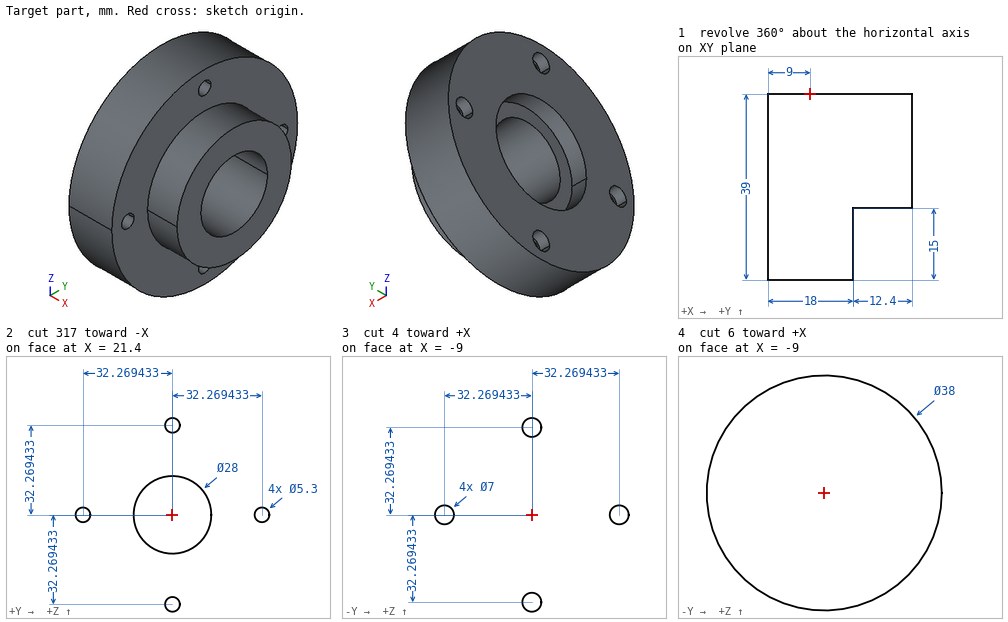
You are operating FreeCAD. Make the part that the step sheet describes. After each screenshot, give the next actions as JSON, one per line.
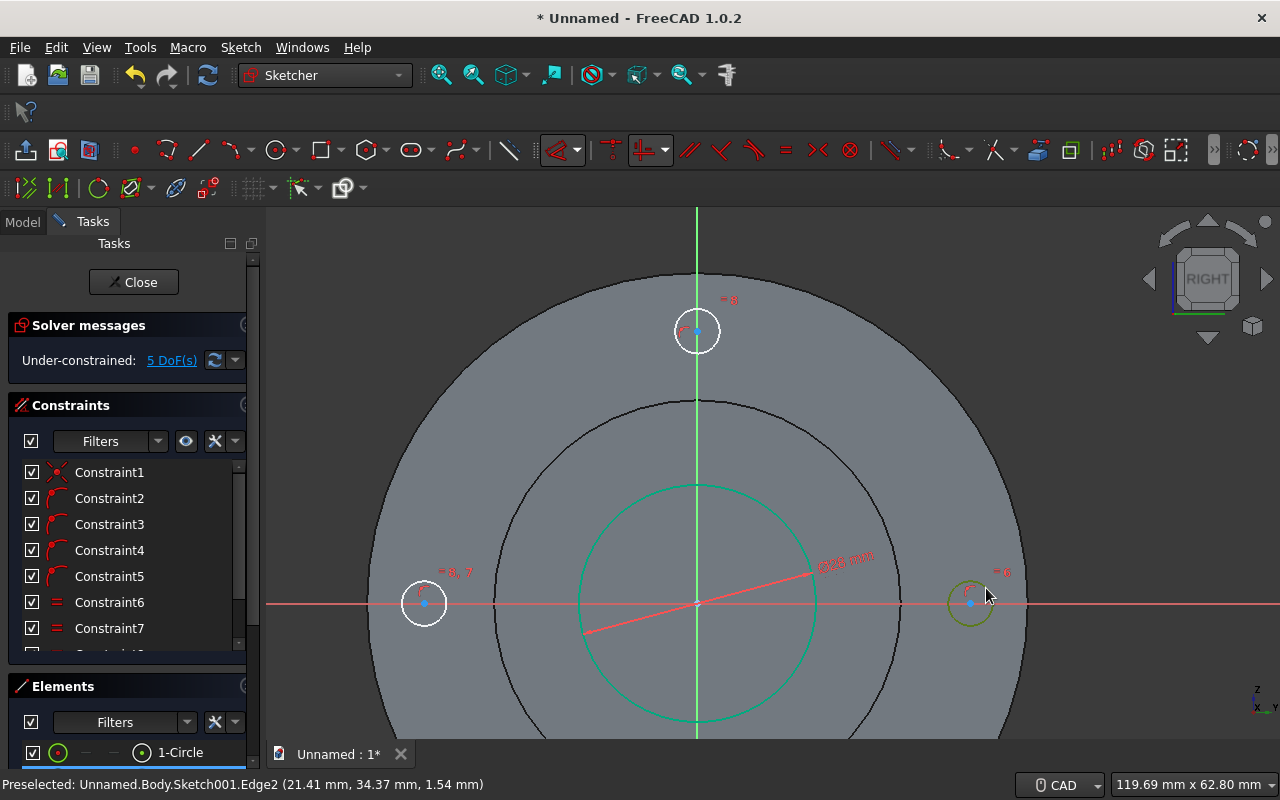
{"action": "key", "text": "k o"}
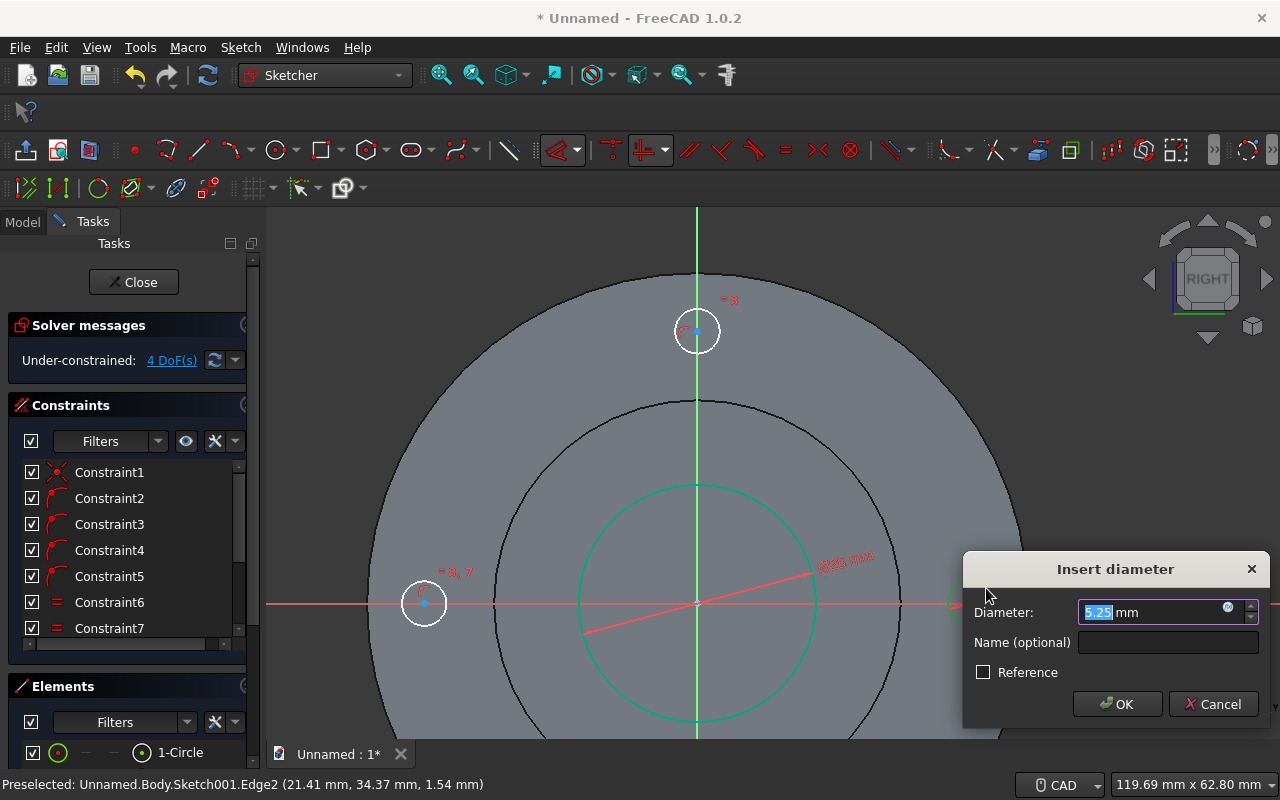
{"action": "type", "text": "5.3"}
{"action": "key", "text": "Return"}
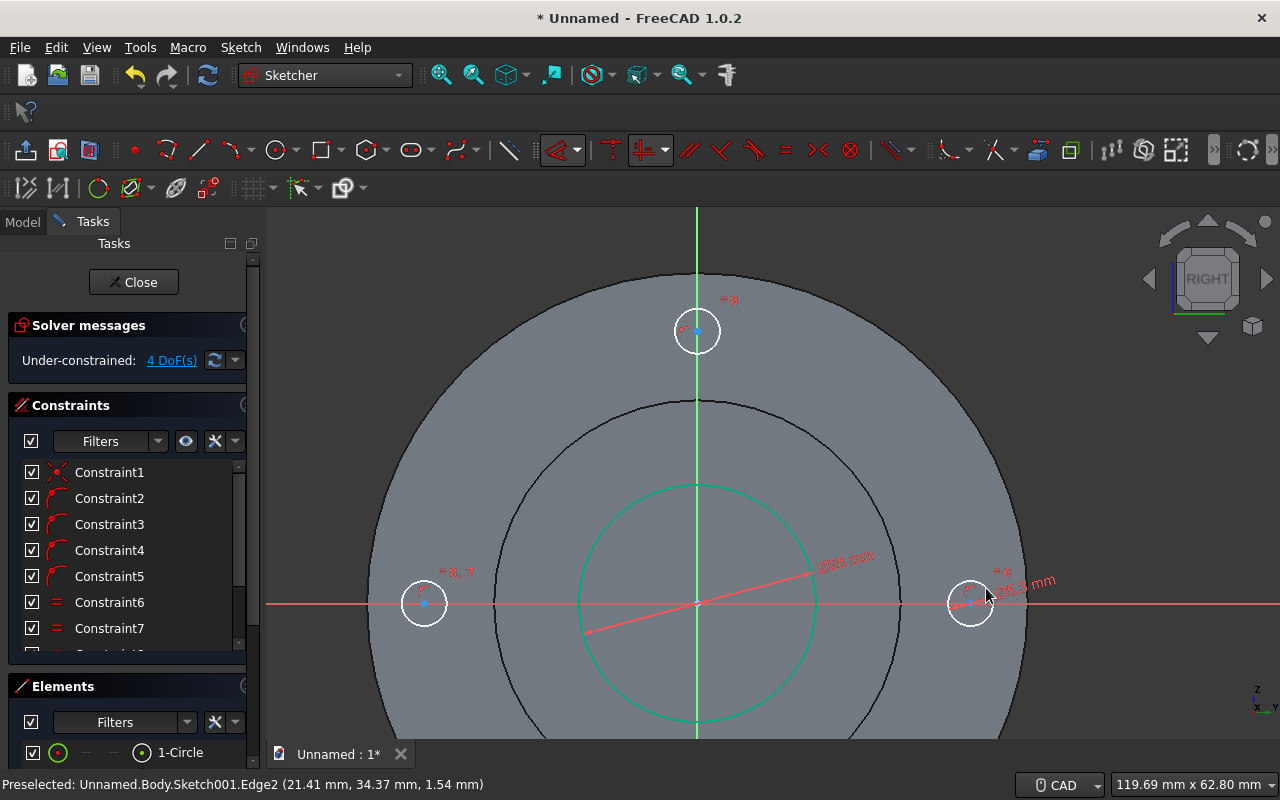
{"action": "left_click", "coordinate": [971, 604]}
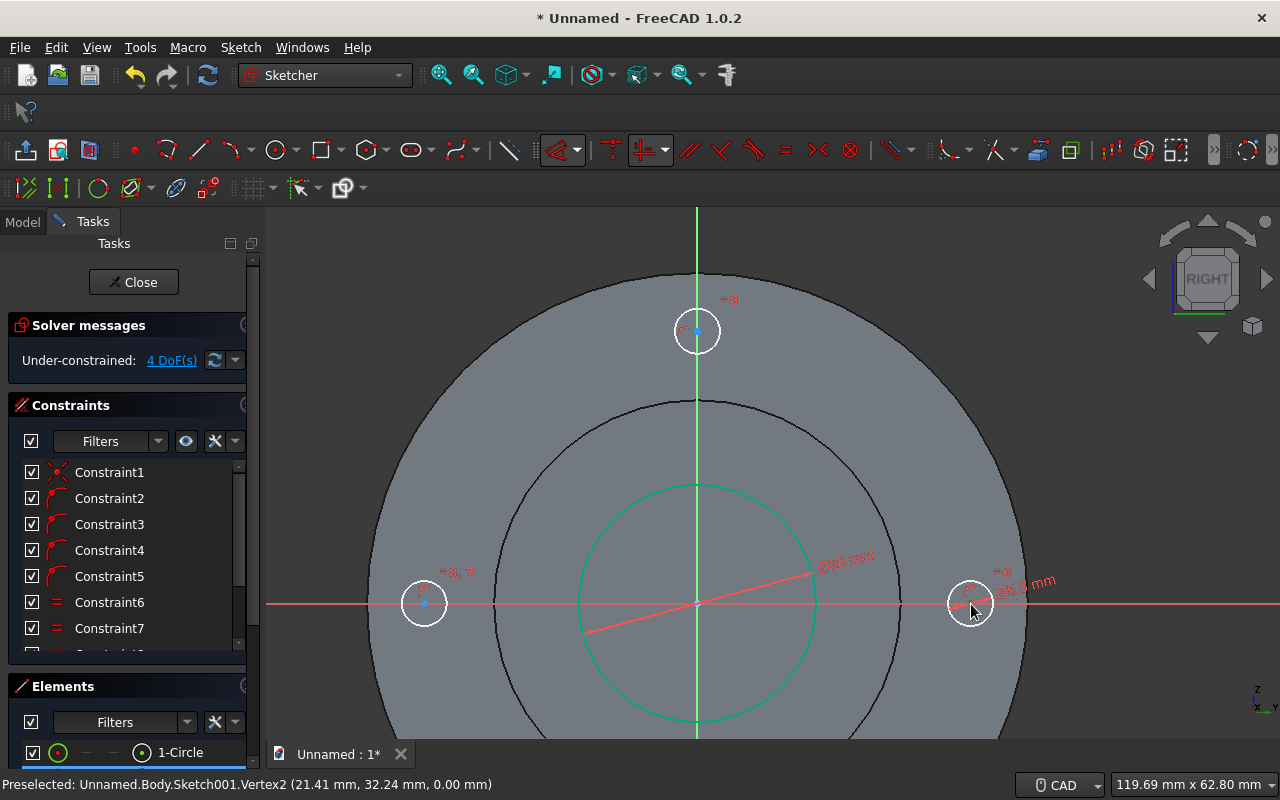
{"action": "left_click", "coordinate": [580, 150]}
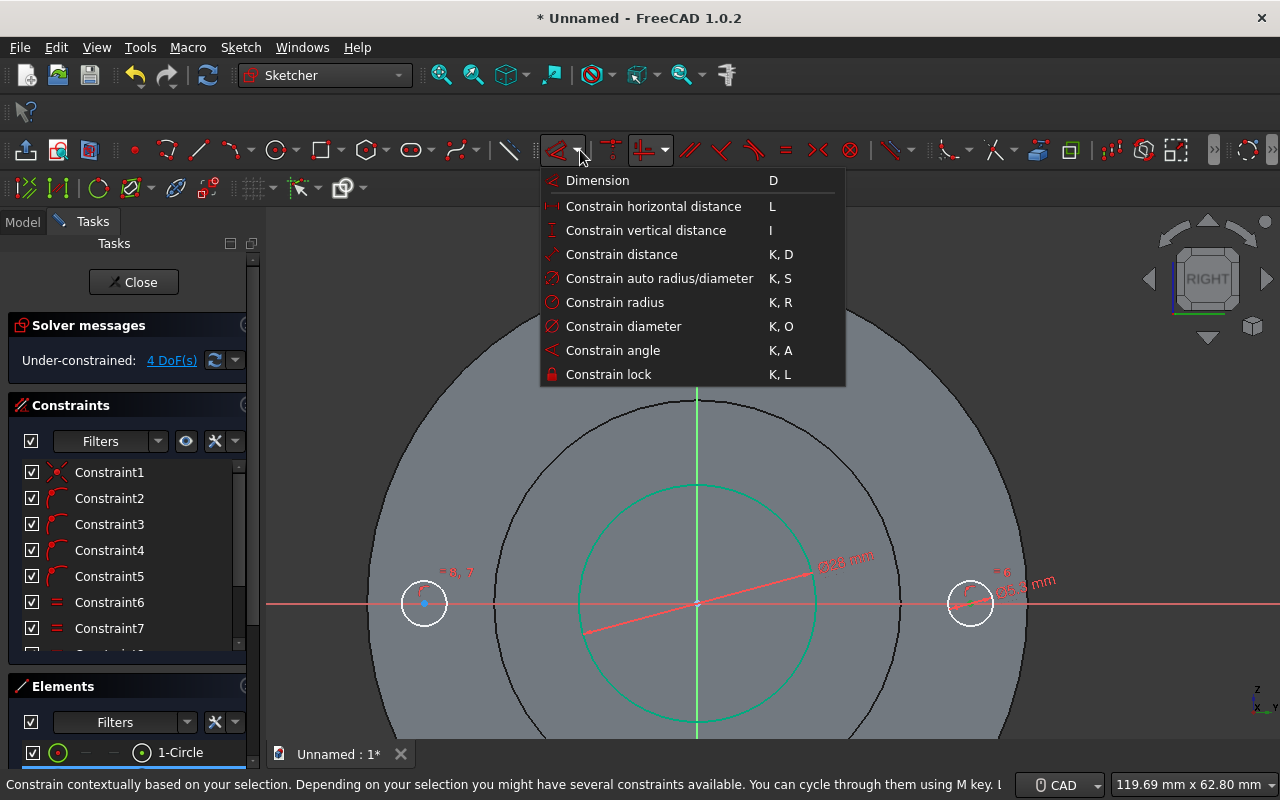
{"action": "left_click", "coordinate": [693, 206]}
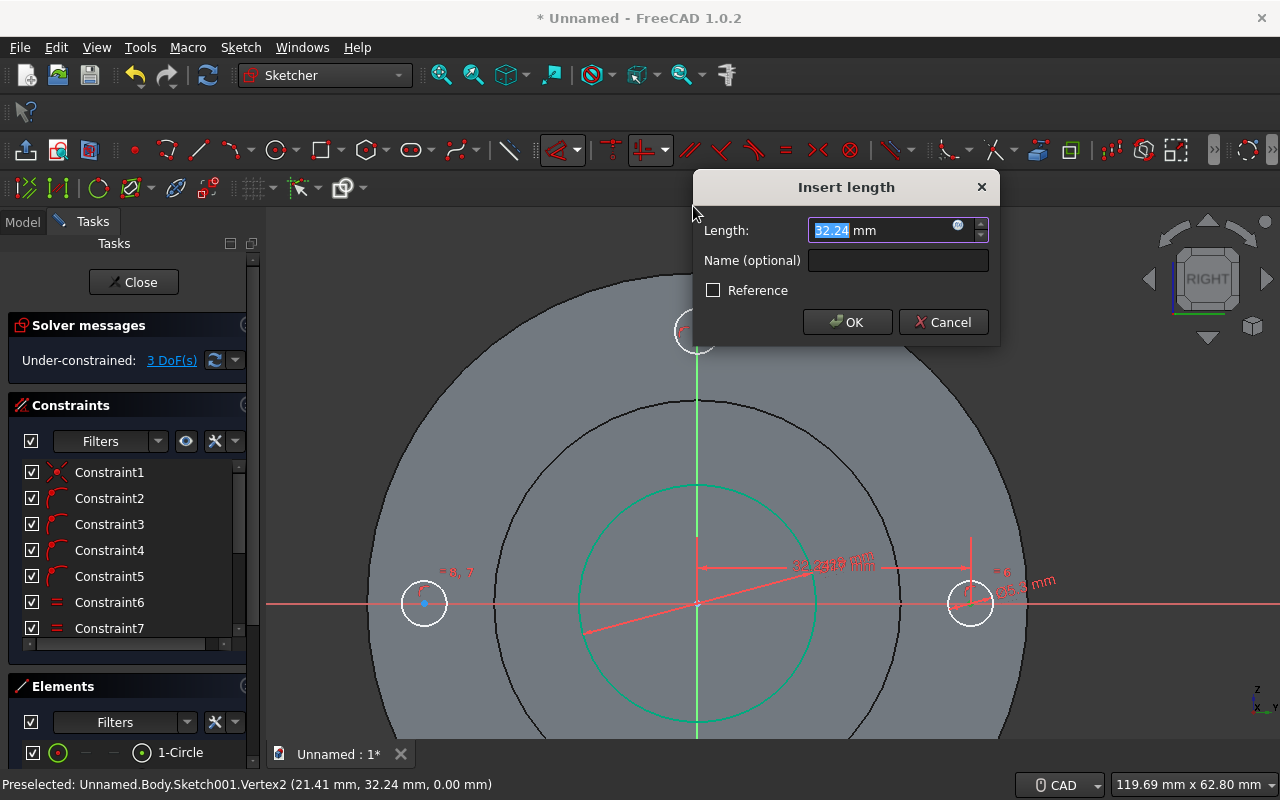
{"action": "type", "text": "32.269433"}
{"action": "key", "text": "Return"}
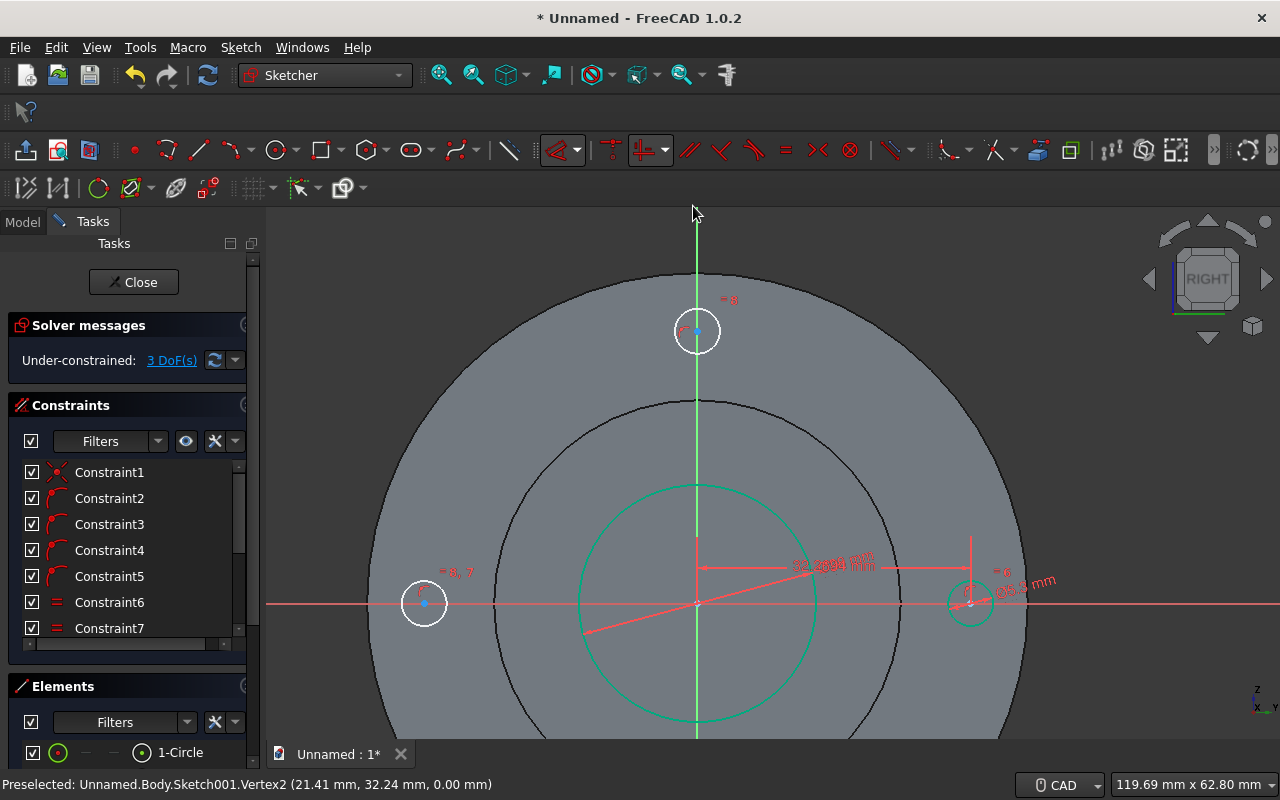
{"action": "scroll", "coordinate": [713, 314], "scroll_direction": "down", "scroll_amount": 3}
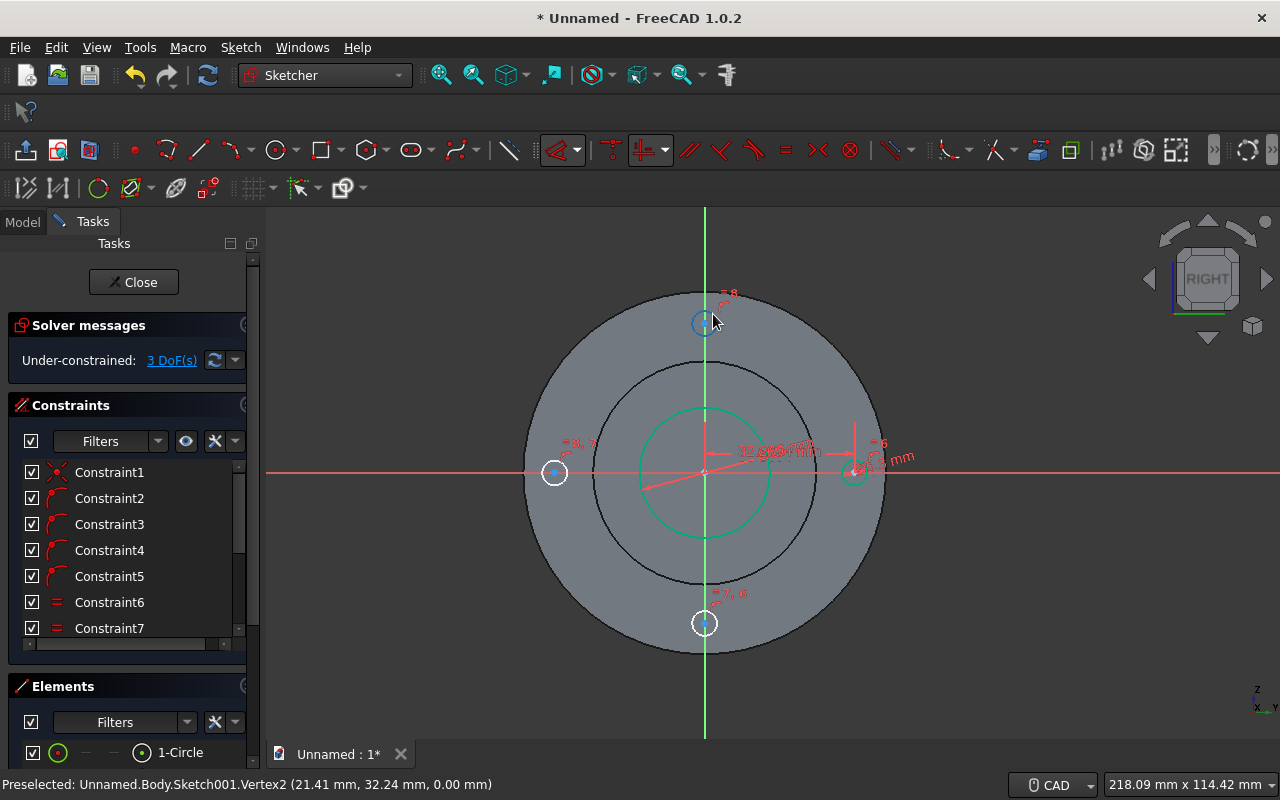
{"action": "left_click", "coordinate": [705, 623]}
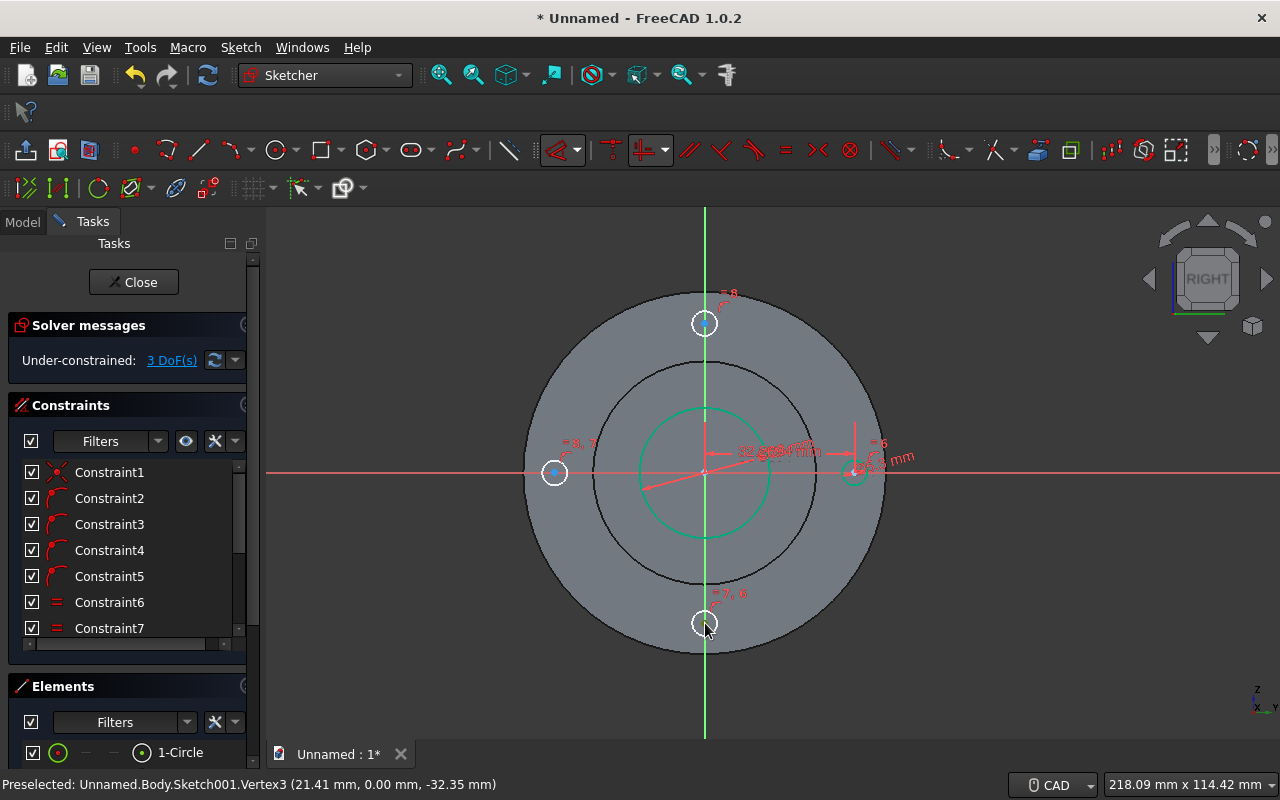
{"action": "key", "text": "i"}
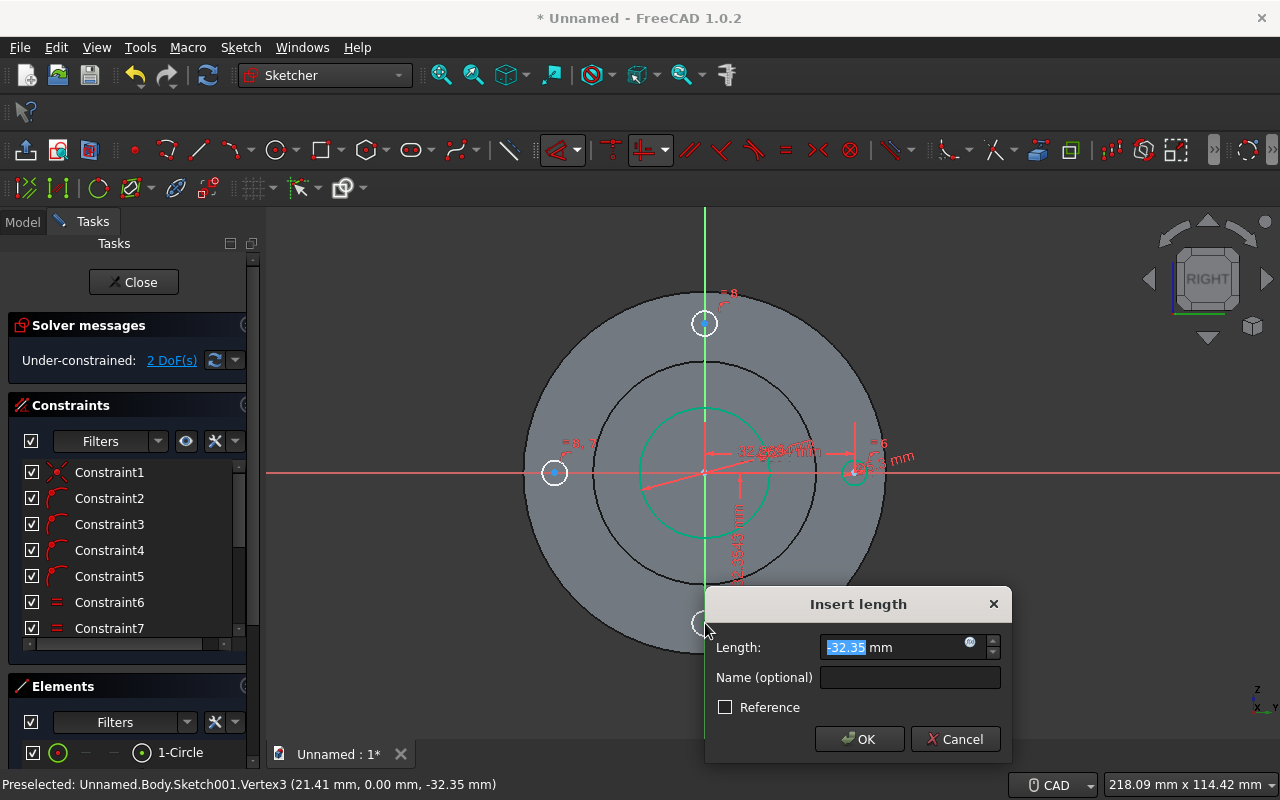
{"action": "type", "text": "-32.269433"}
{"action": "key", "text": "Return"}